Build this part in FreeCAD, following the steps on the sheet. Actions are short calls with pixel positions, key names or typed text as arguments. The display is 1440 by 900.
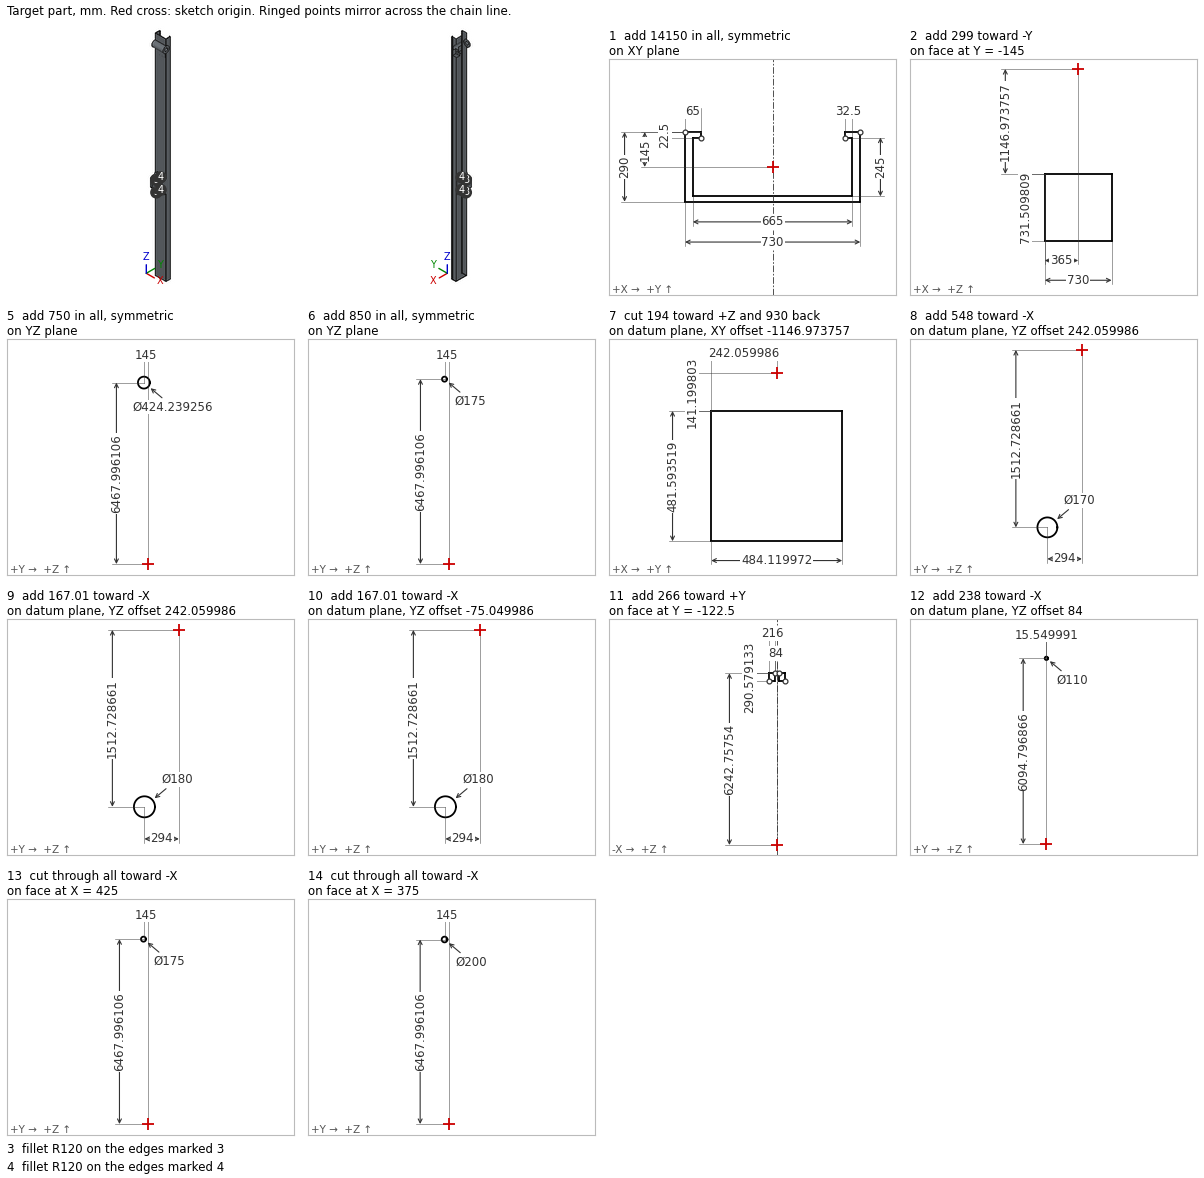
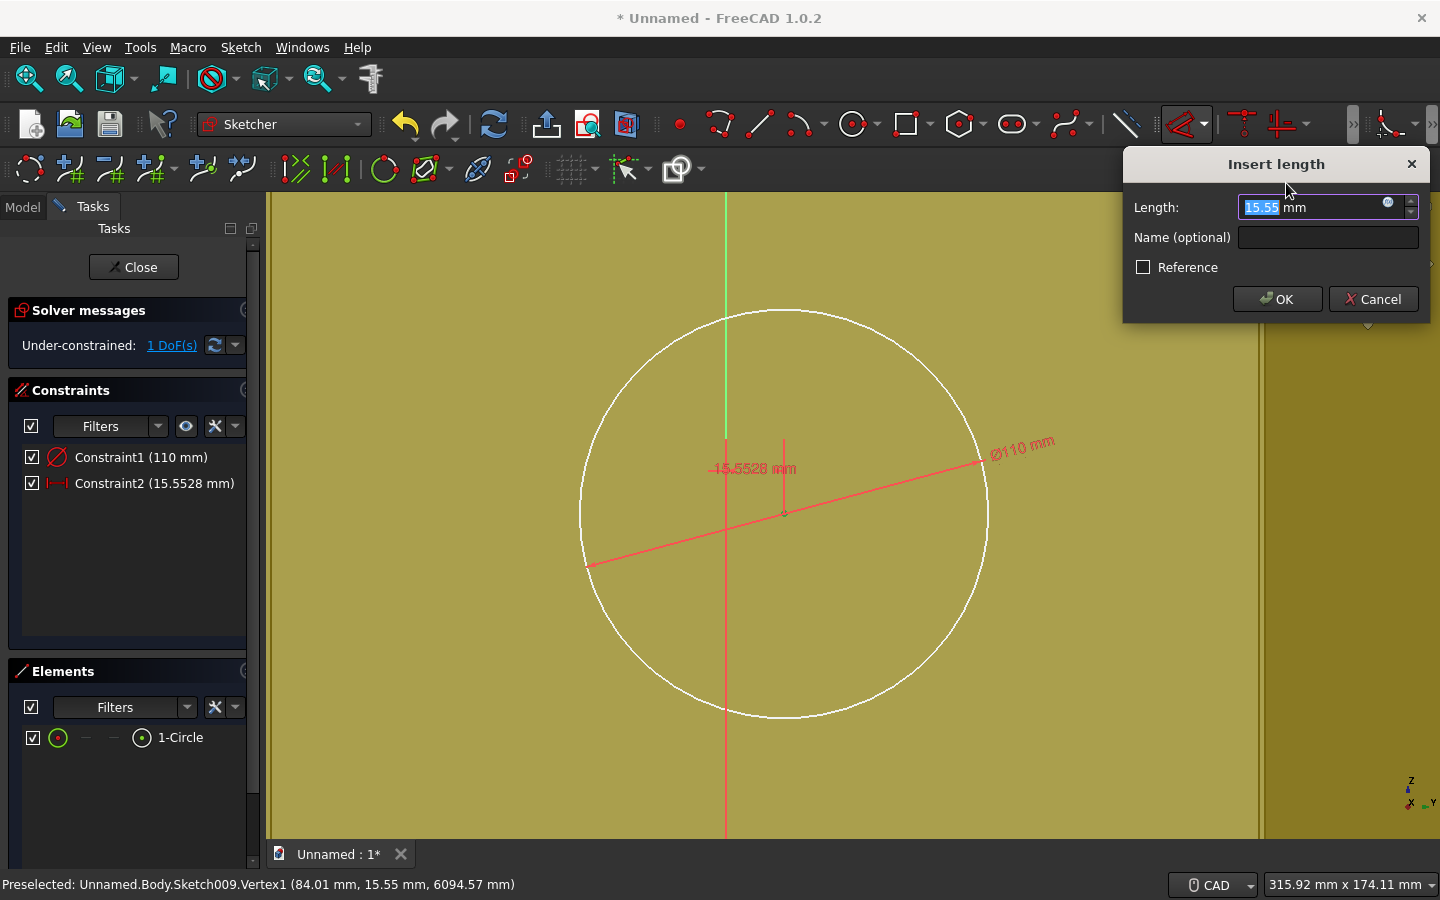
text(15.549991)
key(Return)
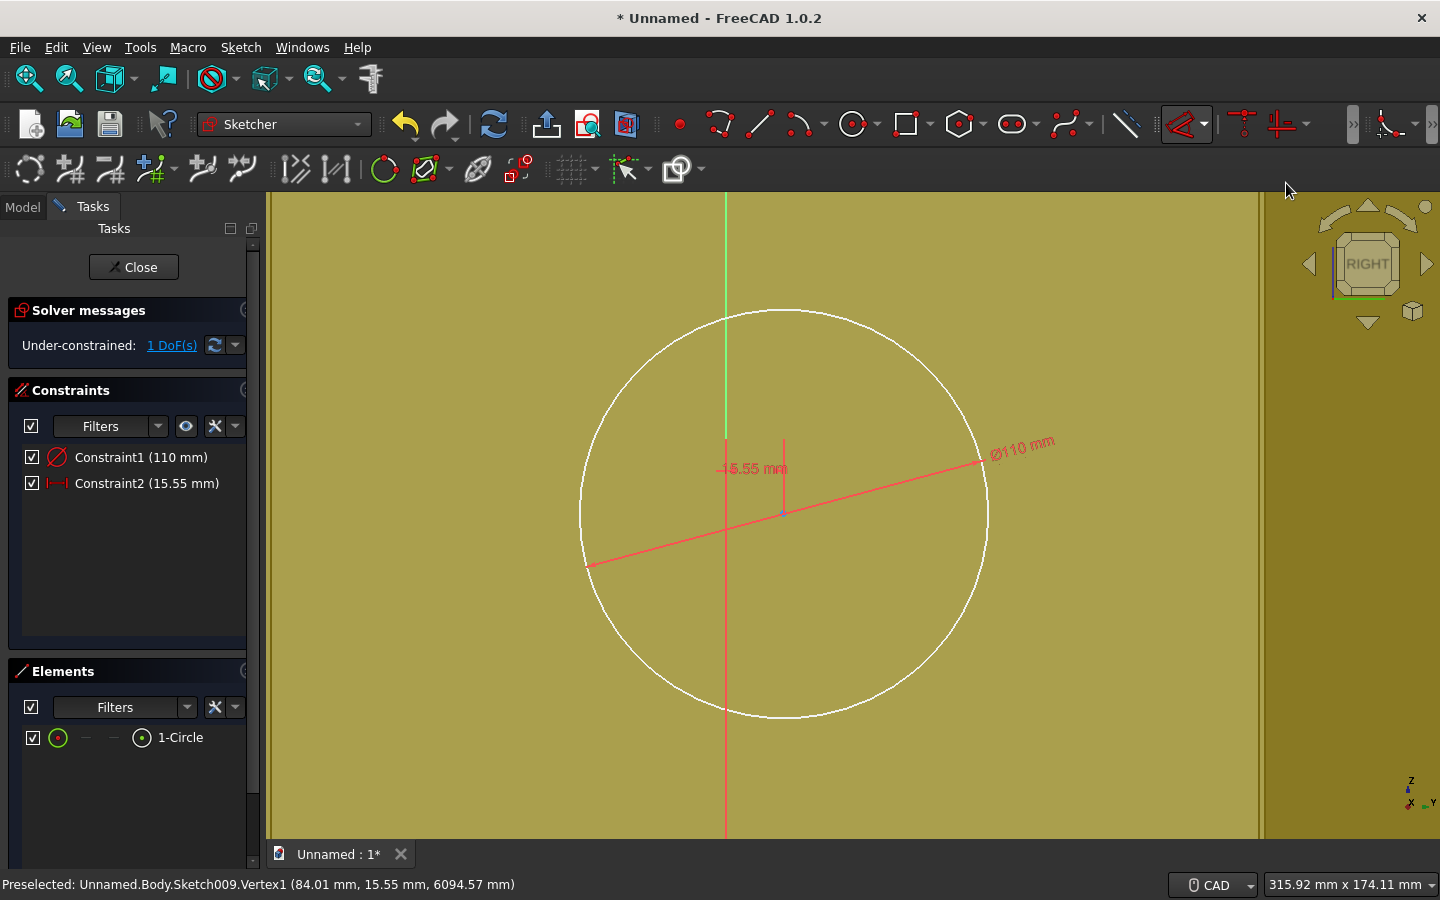
click(784, 514)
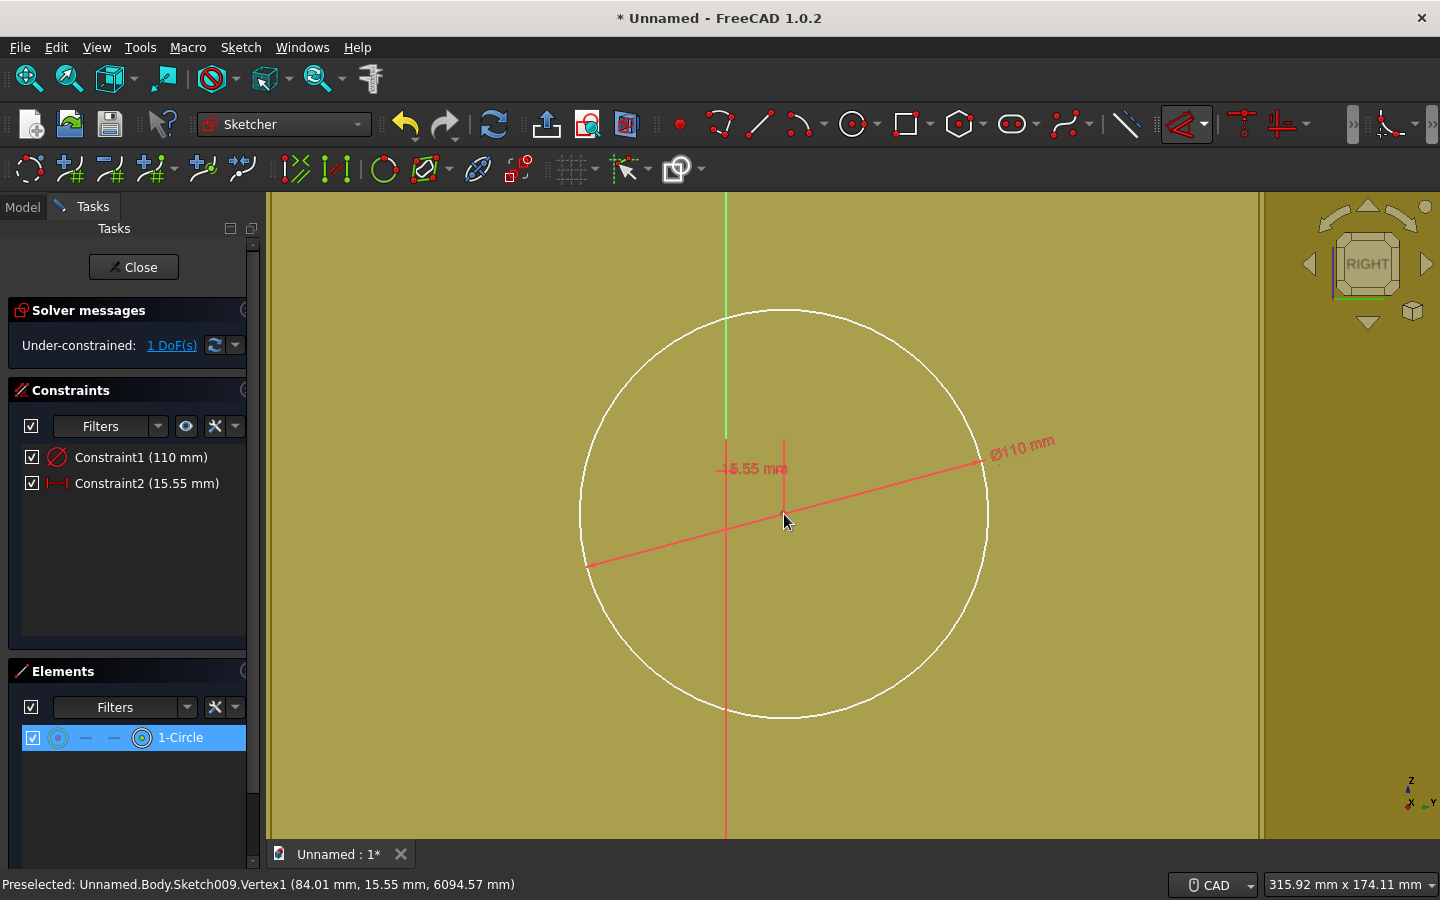
key(i)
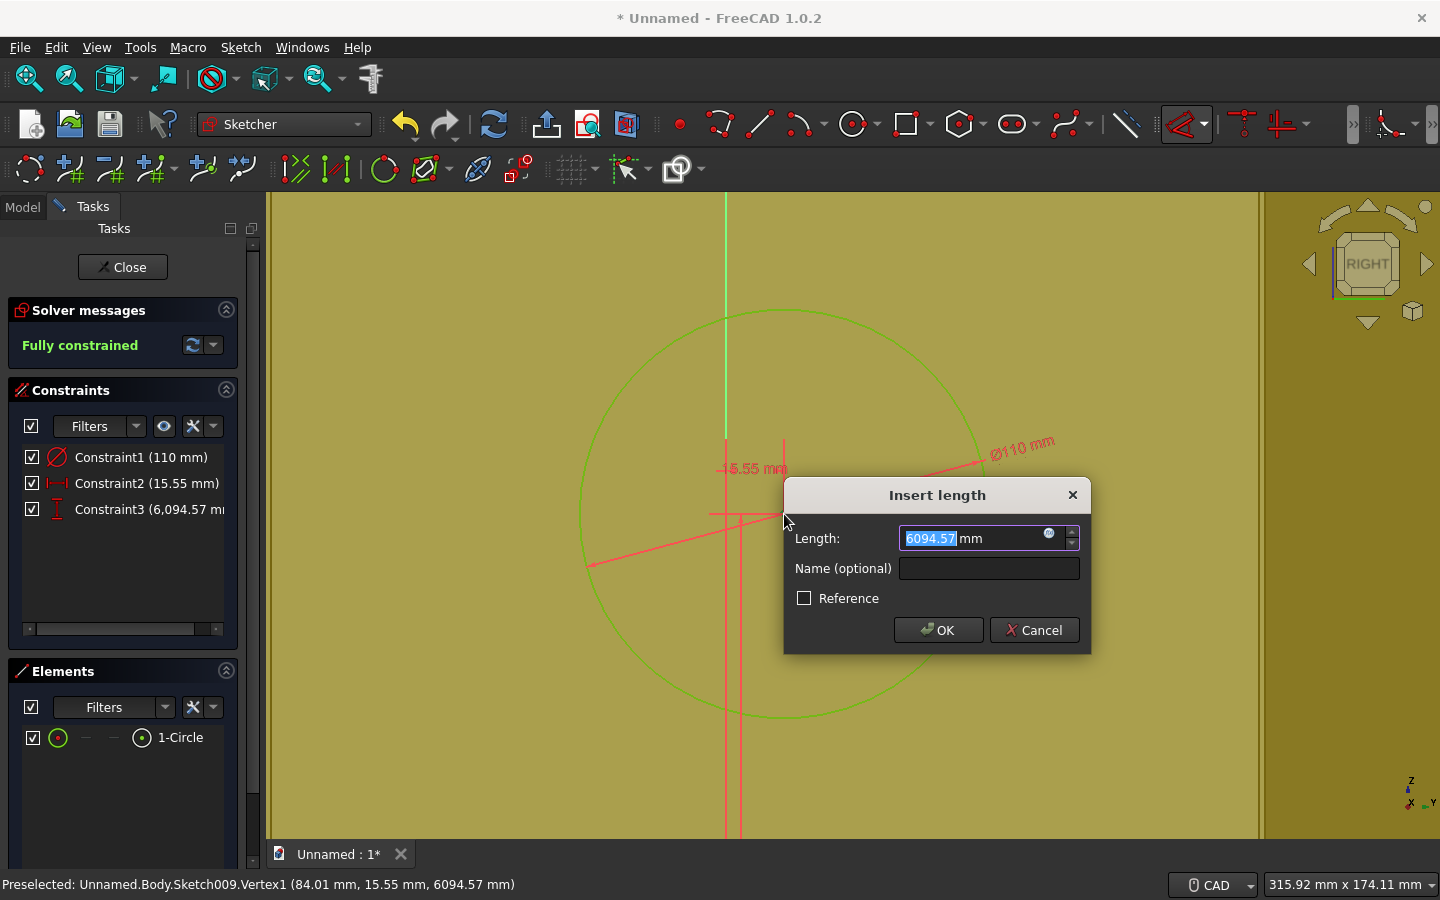
text(6094.796866)
key(Return)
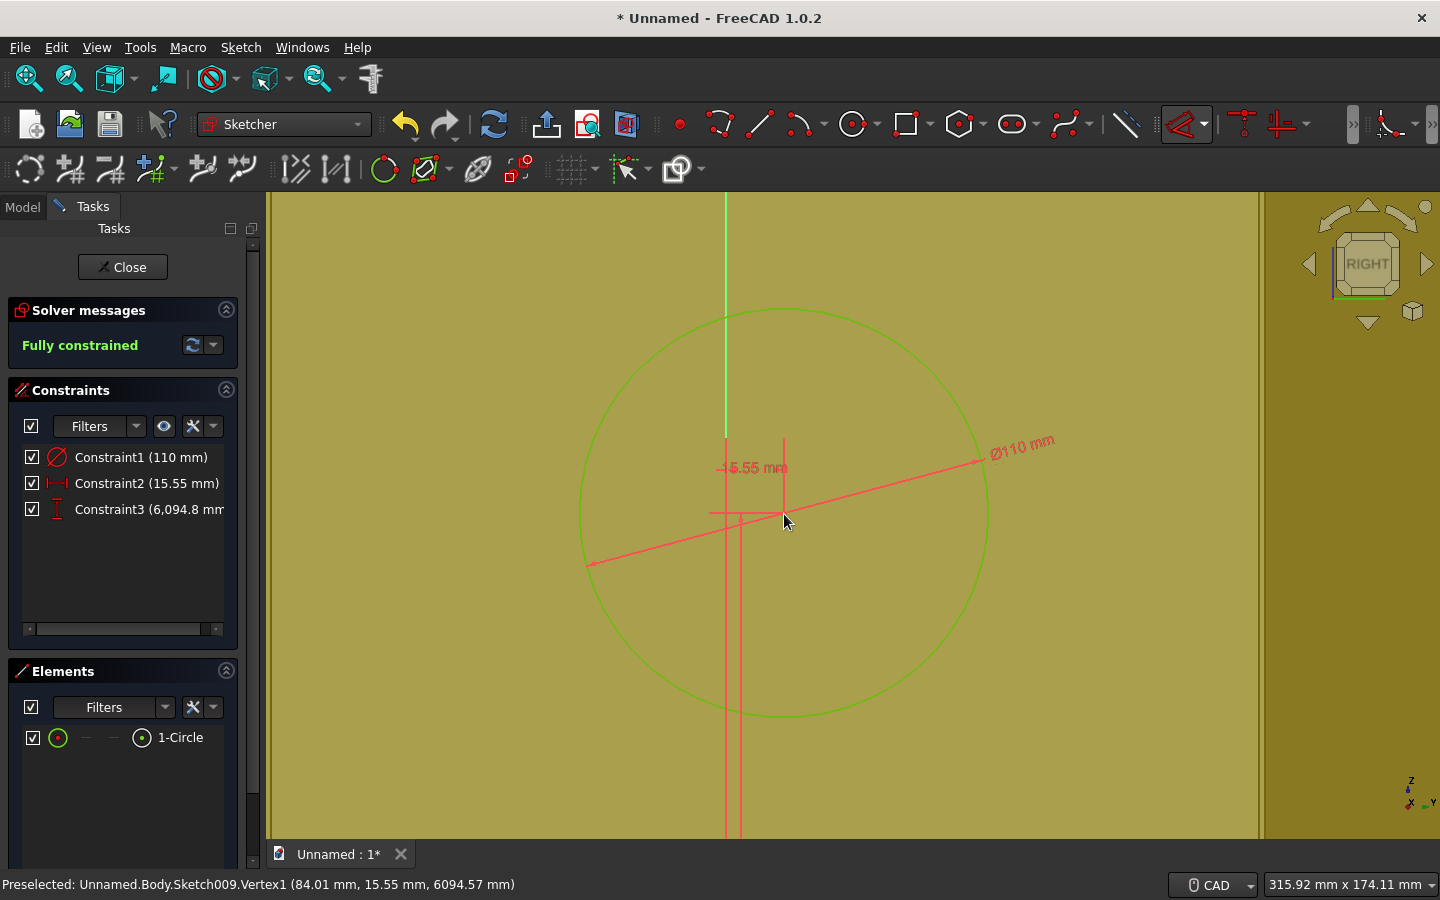
click(123, 267)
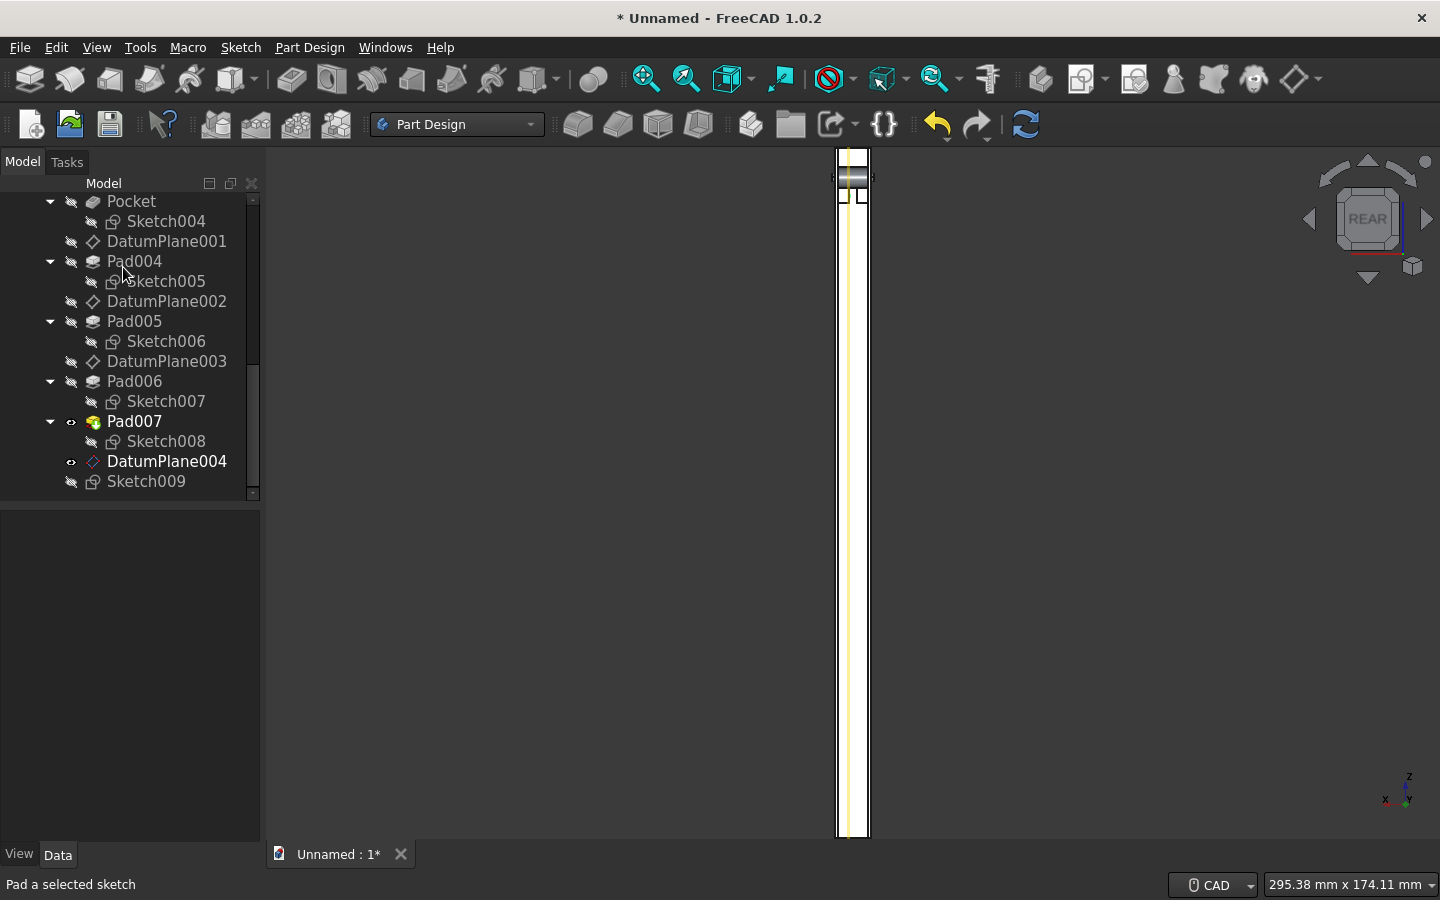
click(30, 80)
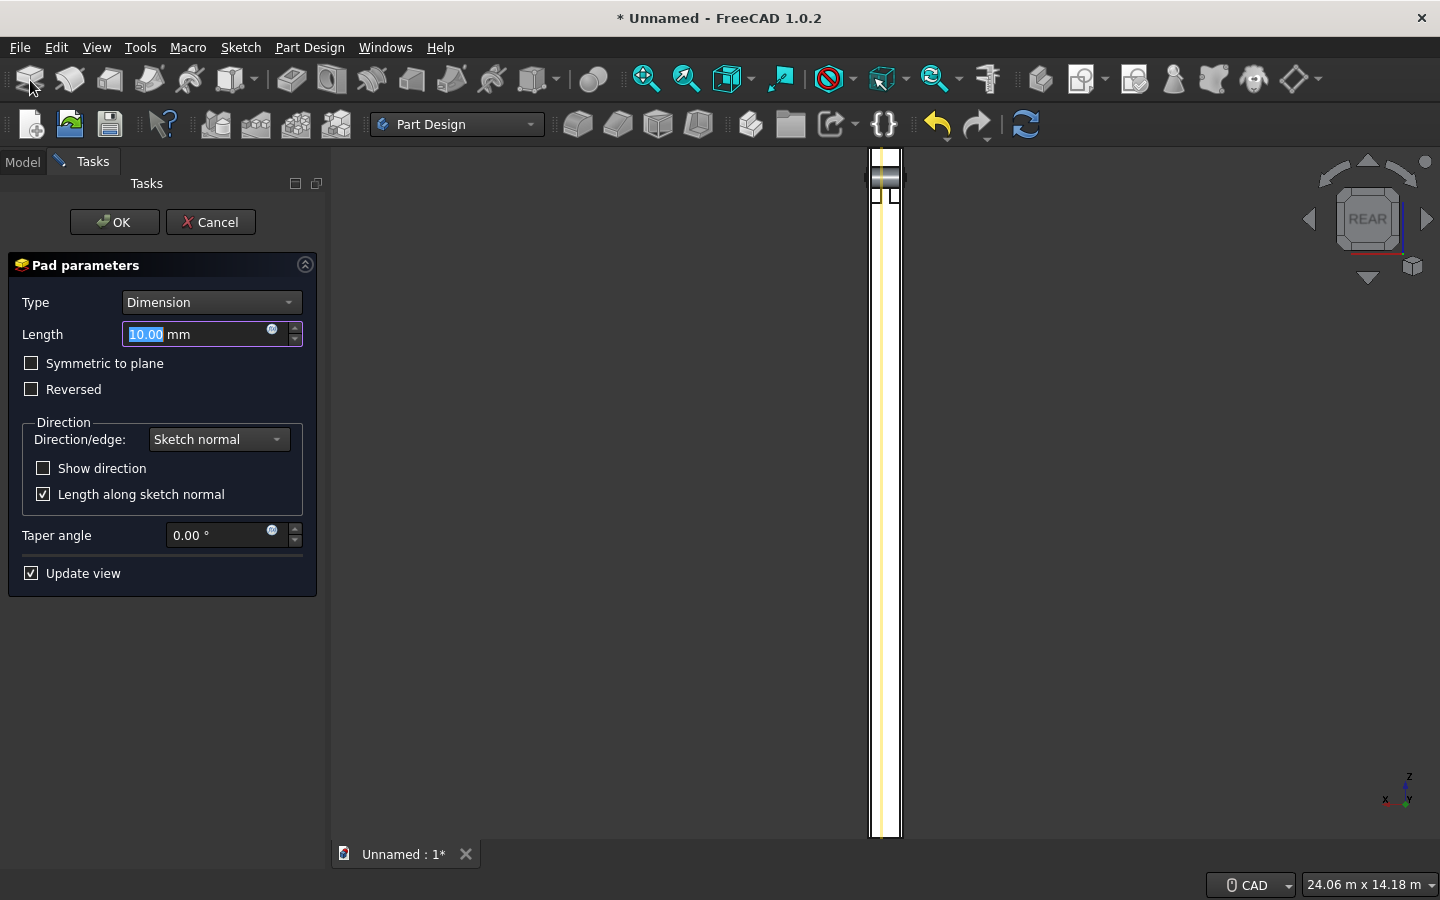
text(238)
key(Tab)